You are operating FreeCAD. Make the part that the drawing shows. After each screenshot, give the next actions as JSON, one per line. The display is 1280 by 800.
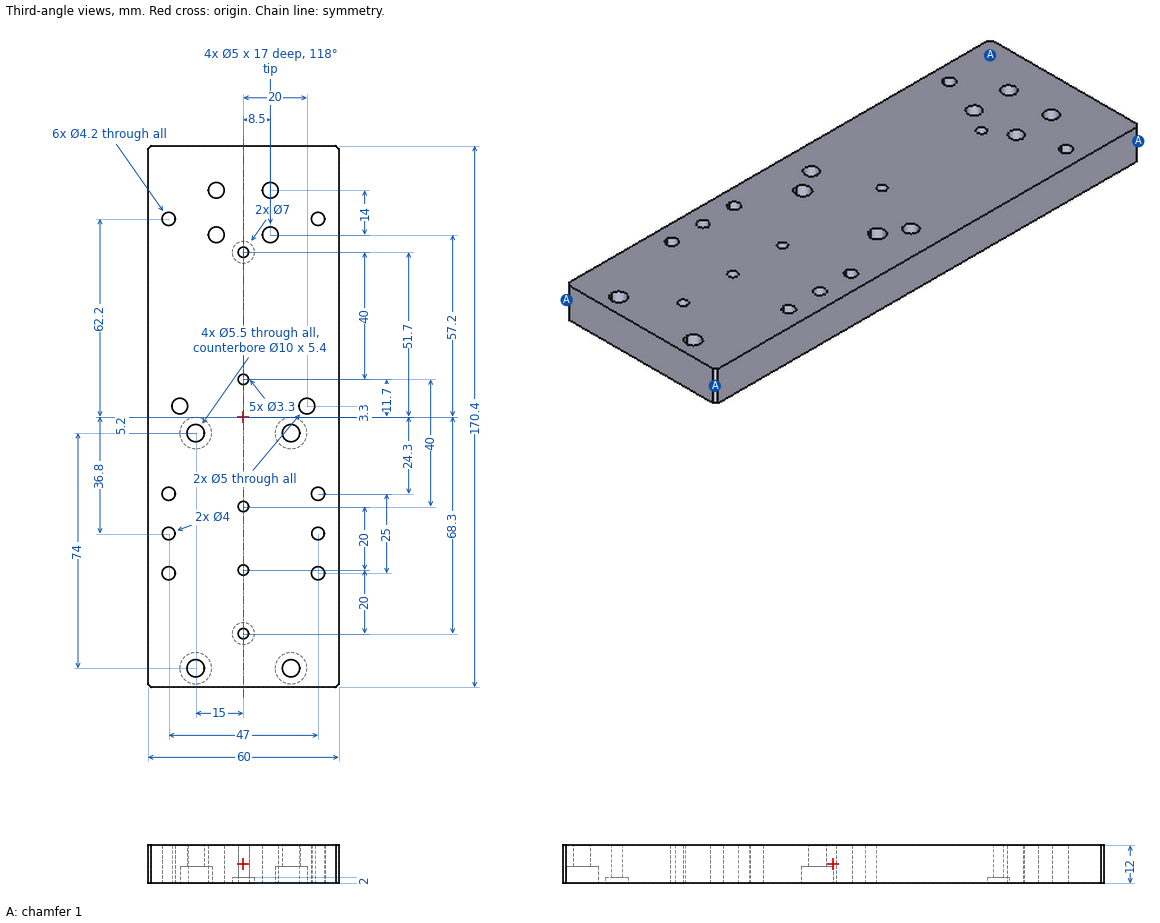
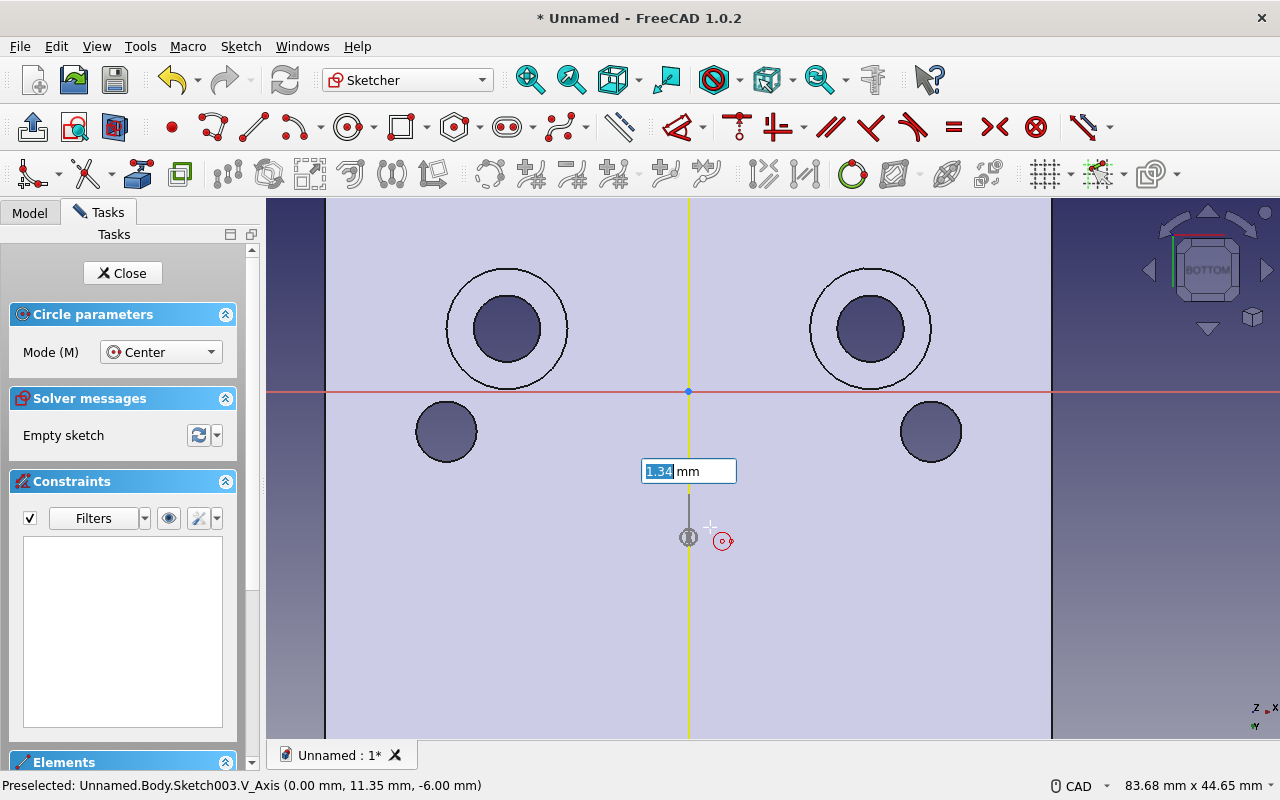
{"action": "left_click", "coordinate": [708, 527]}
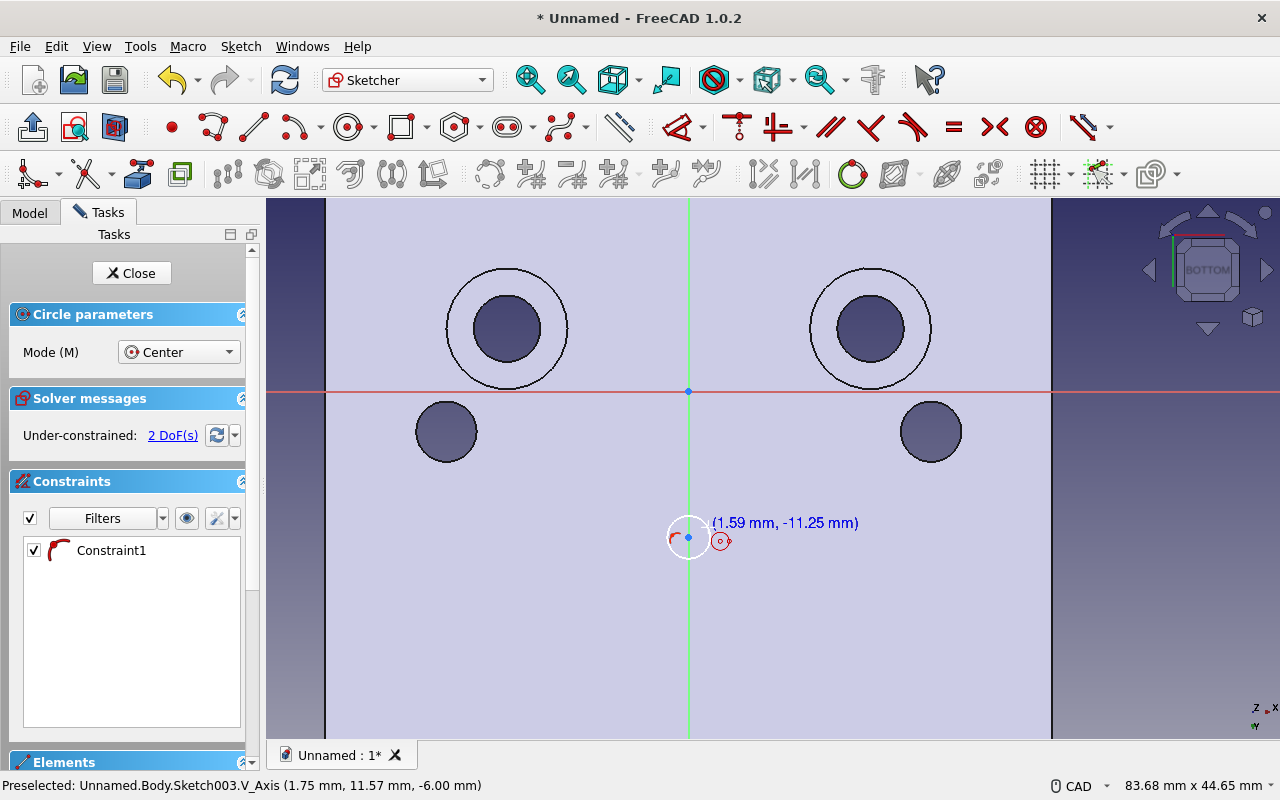
{"action": "scroll", "coordinate": [710, 527], "scroll_direction": "down", "scroll_amount": 7}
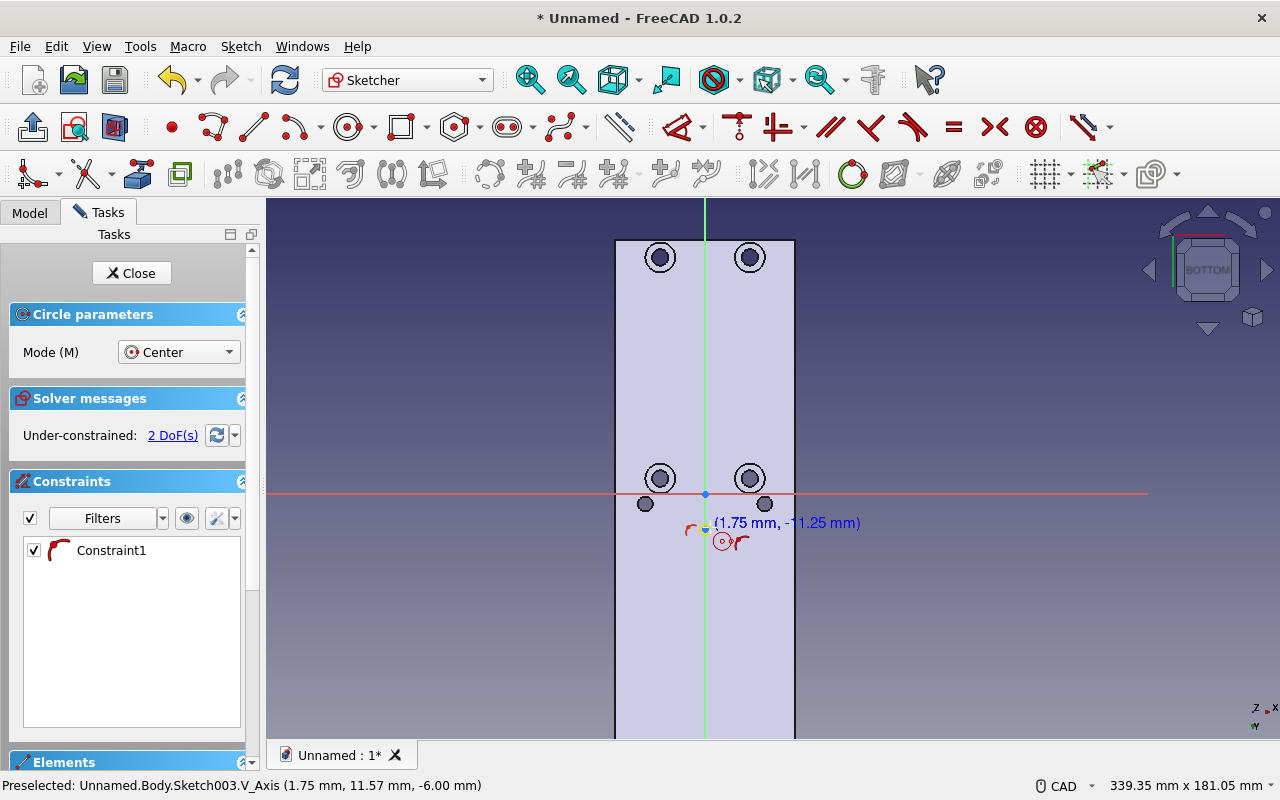
{"action": "scroll", "coordinate": [705, 410], "scroll_direction": "up", "scroll_amount": 8}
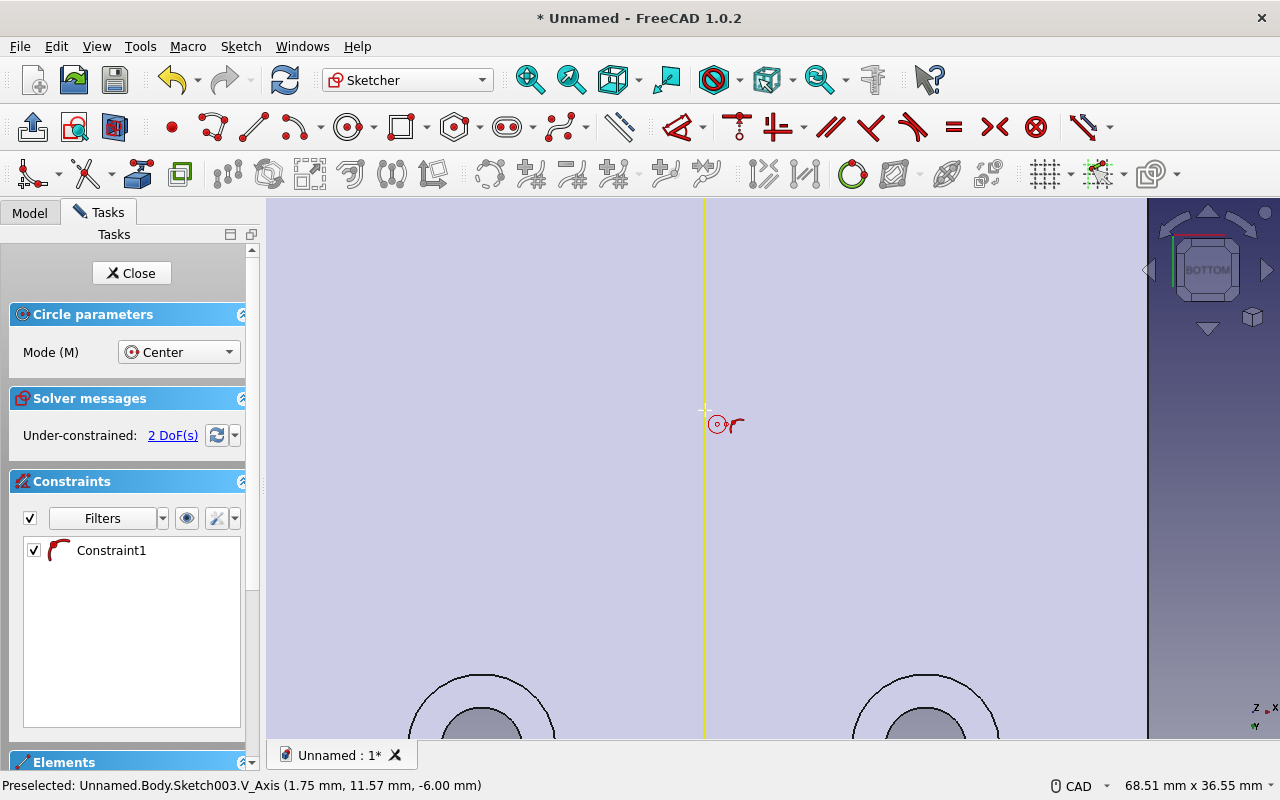
{"action": "scroll", "coordinate": [705, 409], "scroll_direction": "down", "scroll_amount": 8}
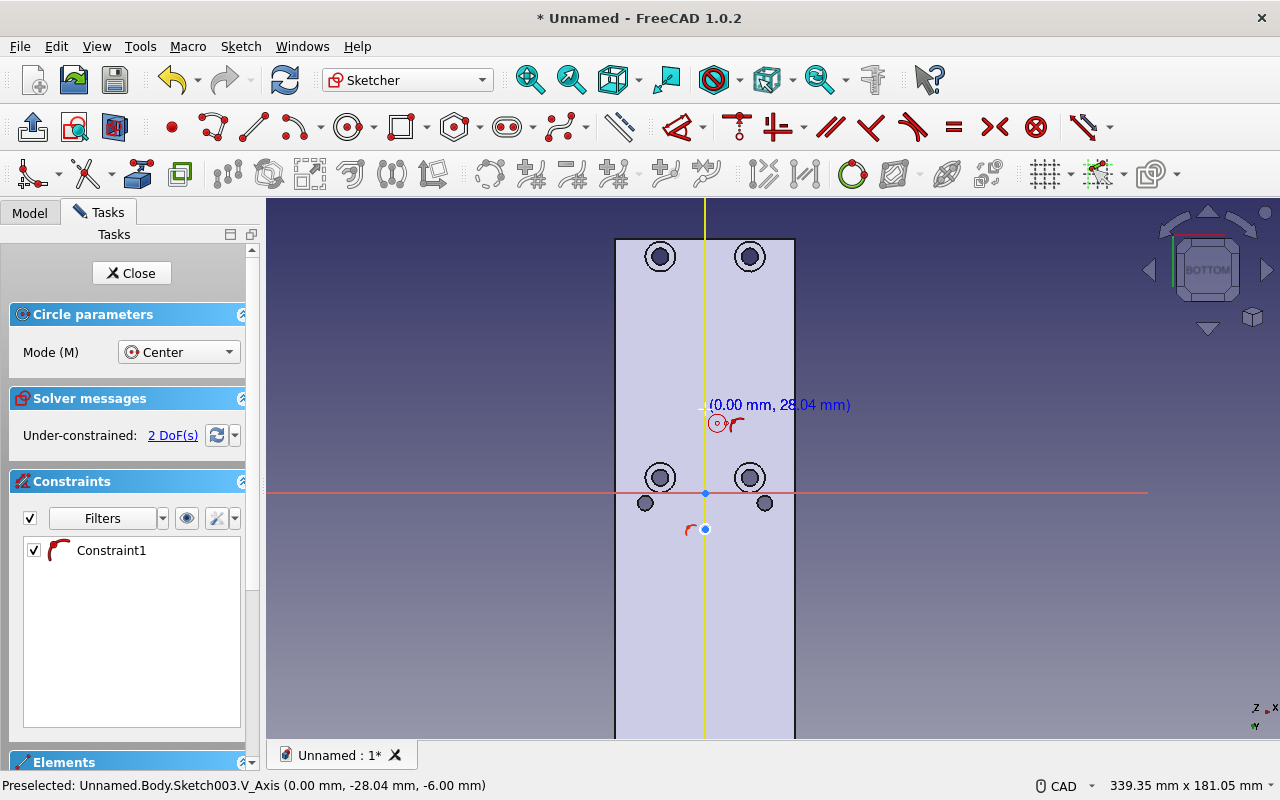
{"action": "left_click", "coordinate": [705, 409]}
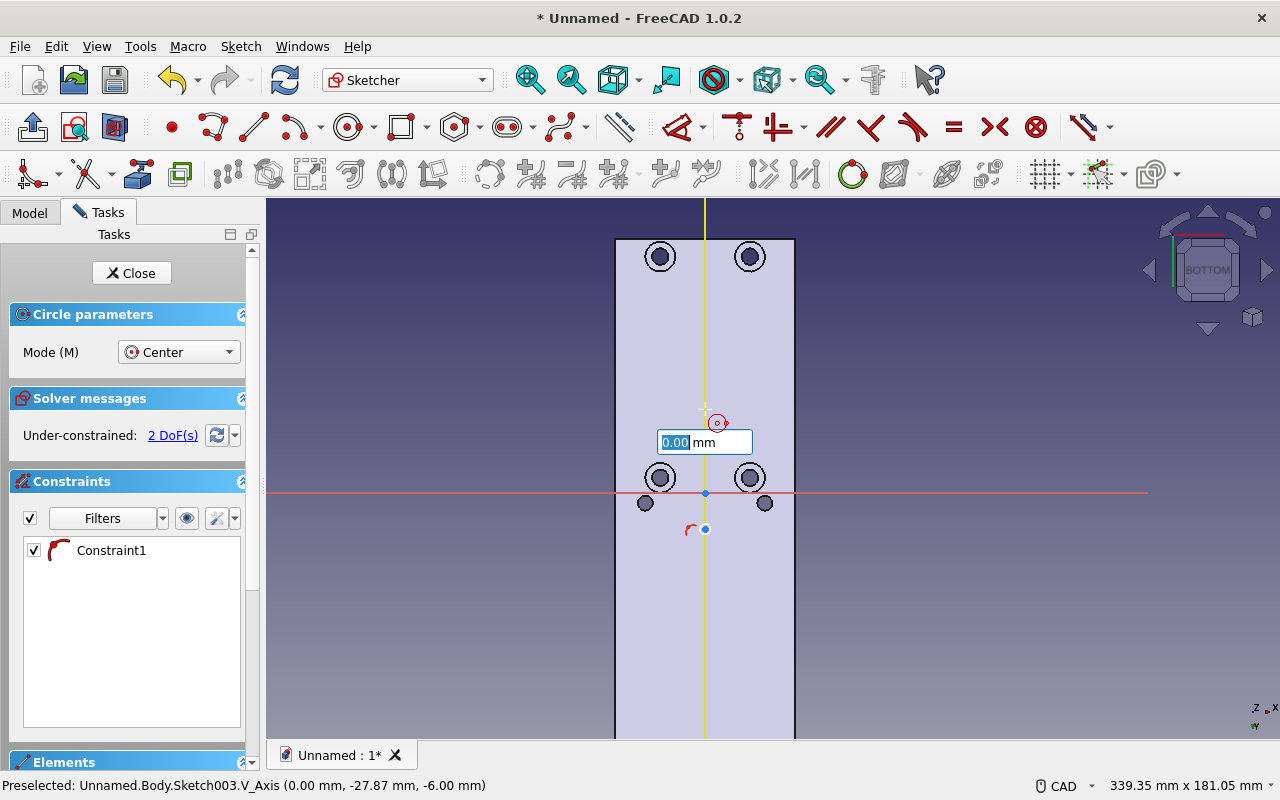
{"action": "scroll", "coordinate": [710, 407], "scroll_direction": "up", "scroll_amount": 7}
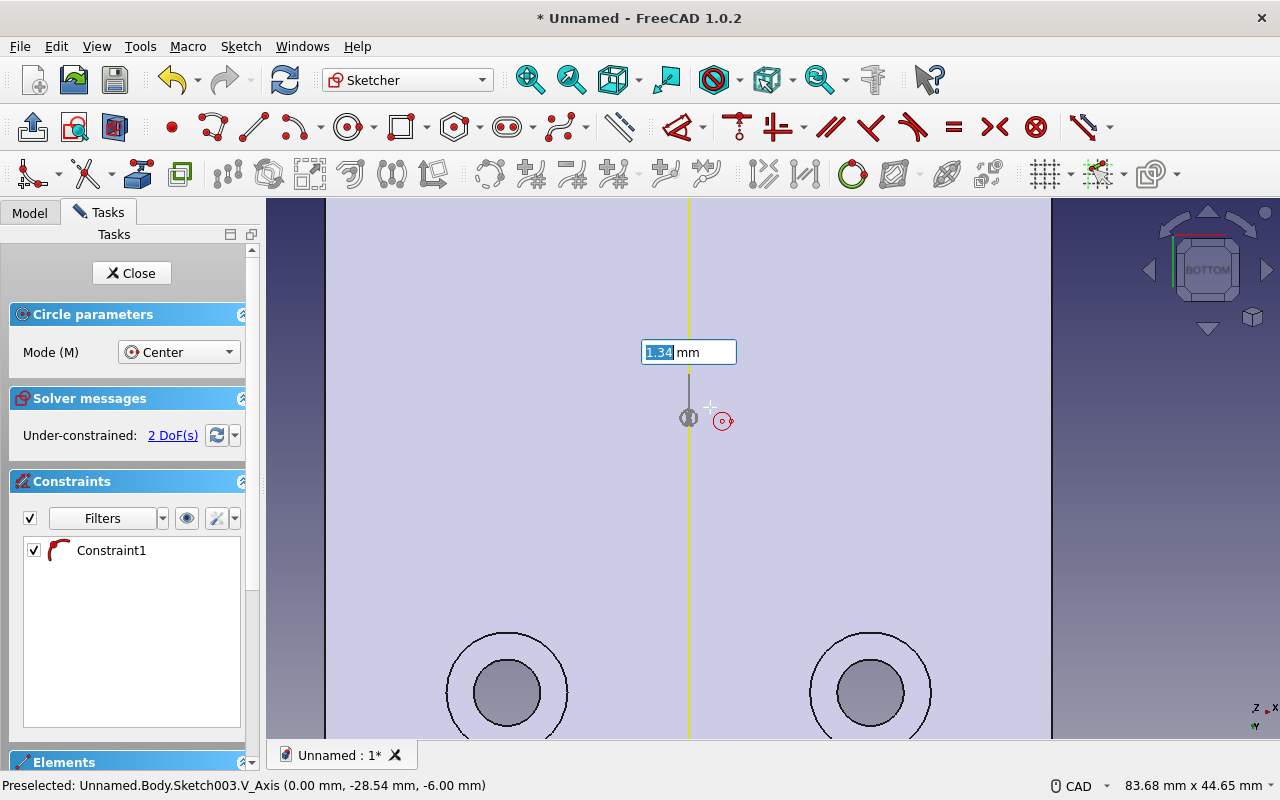
{"action": "left_click", "coordinate": [708, 406]}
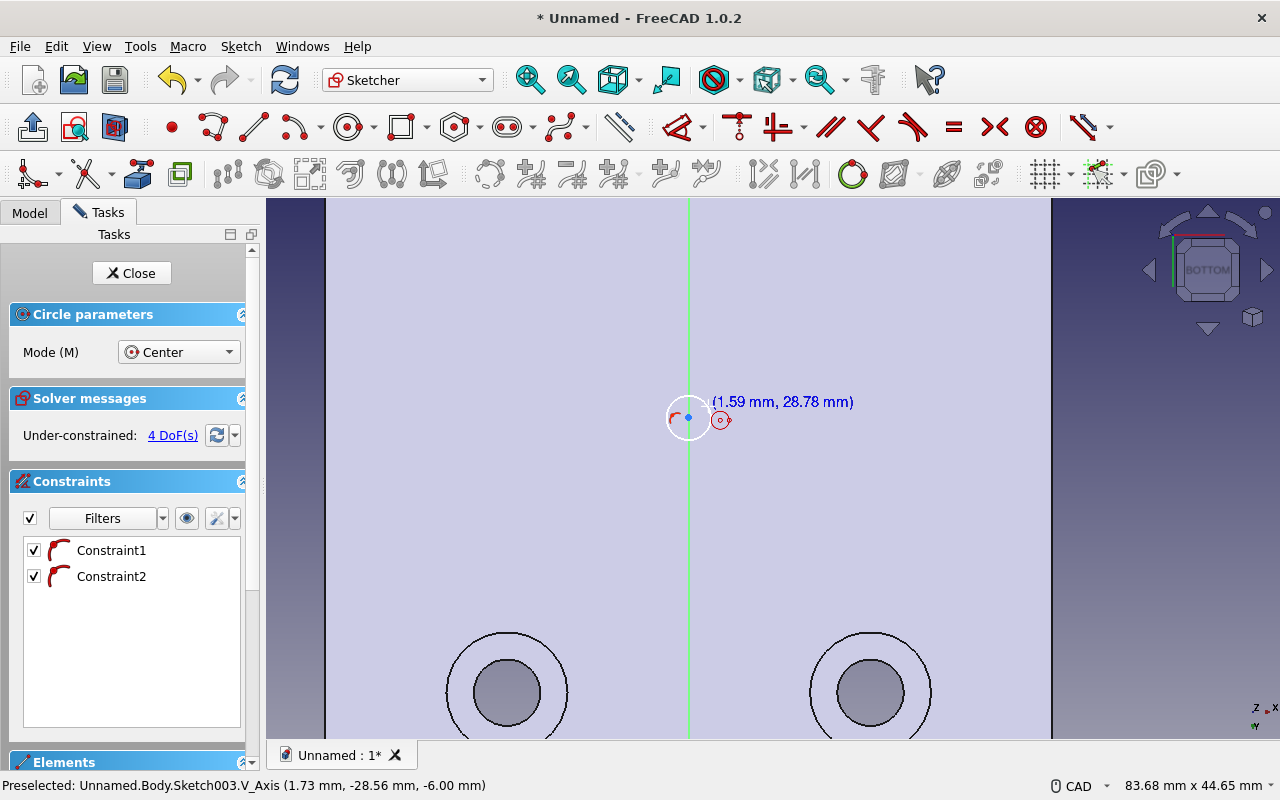
{"action": "scroll", "coordinate": [710, 407], "scroll_direction": "down", "scroll_amount": 7}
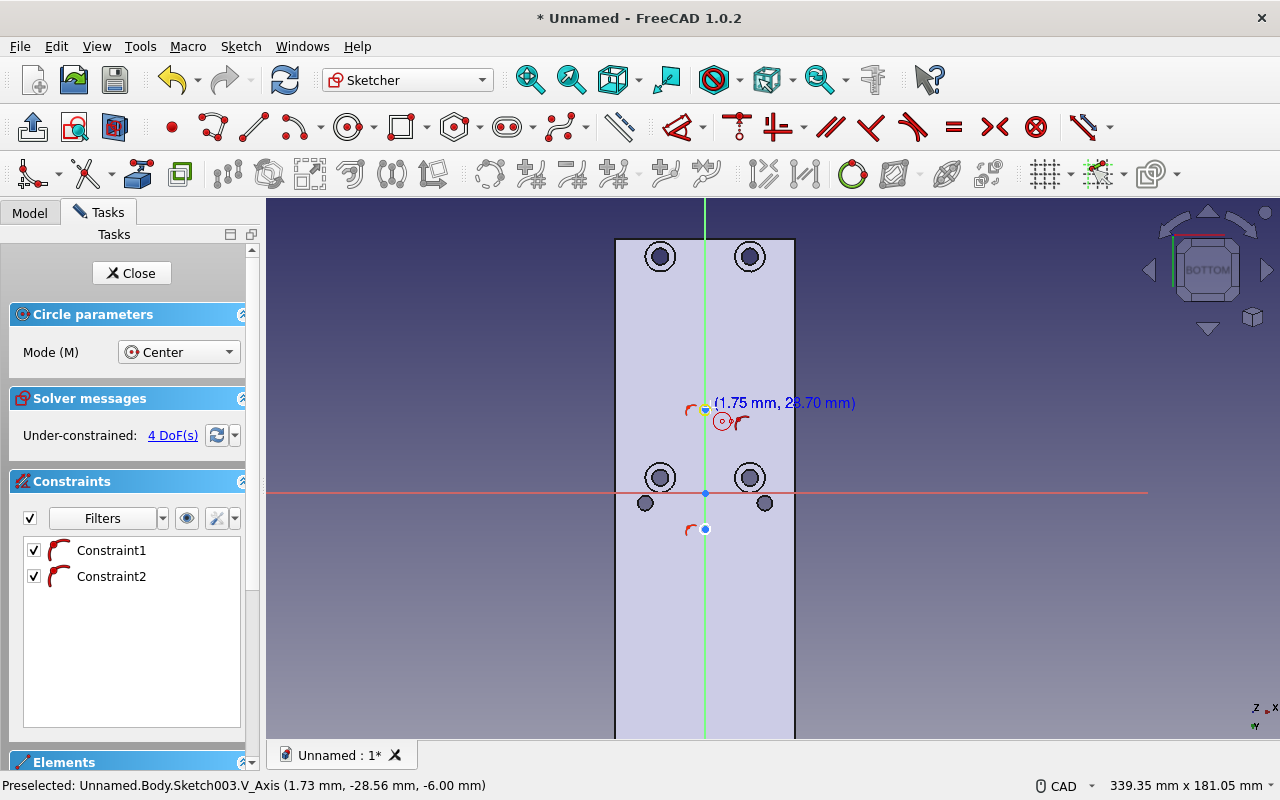
{"action": "scroll", "coordinate": [705, 349], "scroll_direction": "up", "scroll_amount": 8}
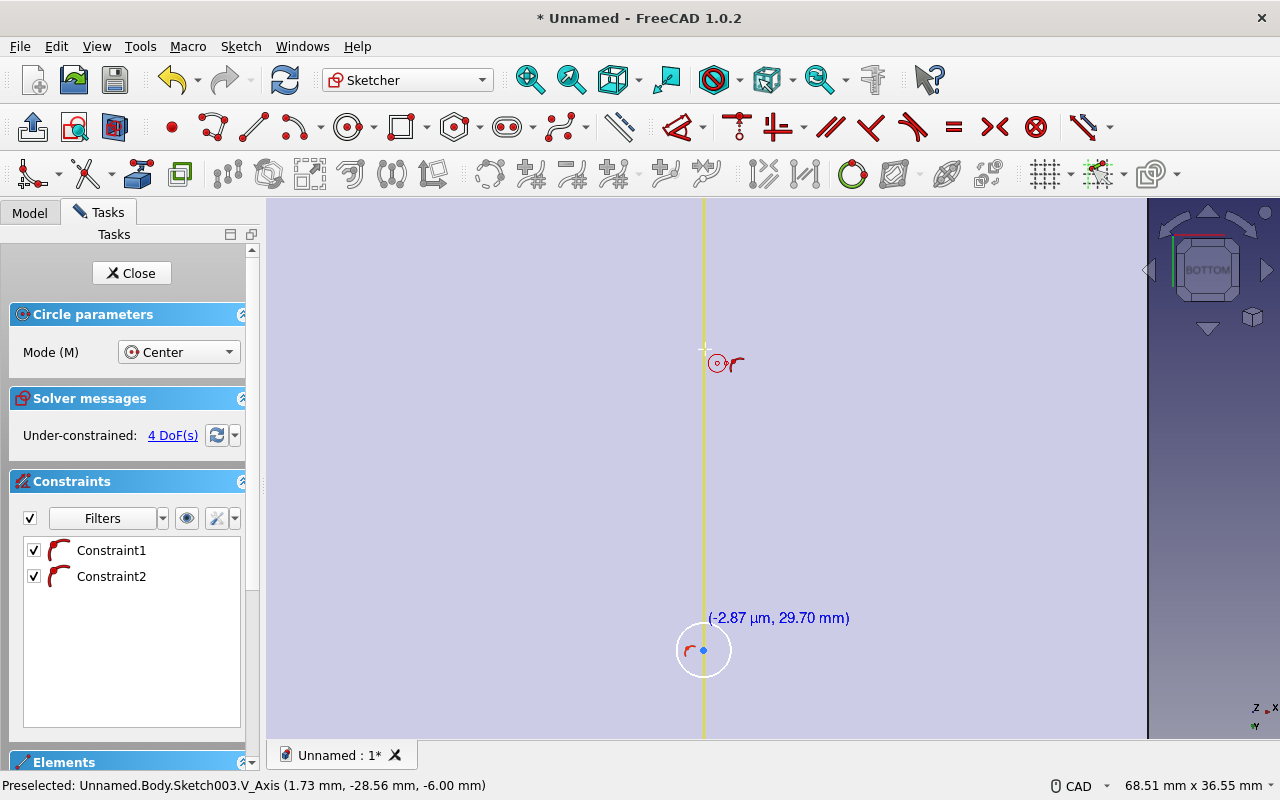
{"action": "scroll", "coordinate": [705, 349], "scroll_direction": "down", "scroll_amount": 8}